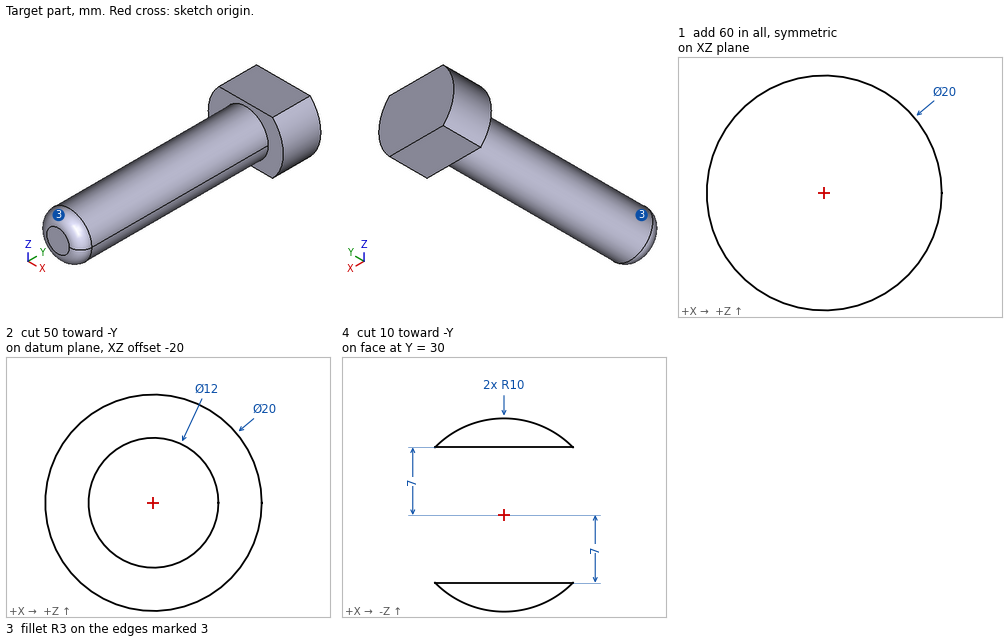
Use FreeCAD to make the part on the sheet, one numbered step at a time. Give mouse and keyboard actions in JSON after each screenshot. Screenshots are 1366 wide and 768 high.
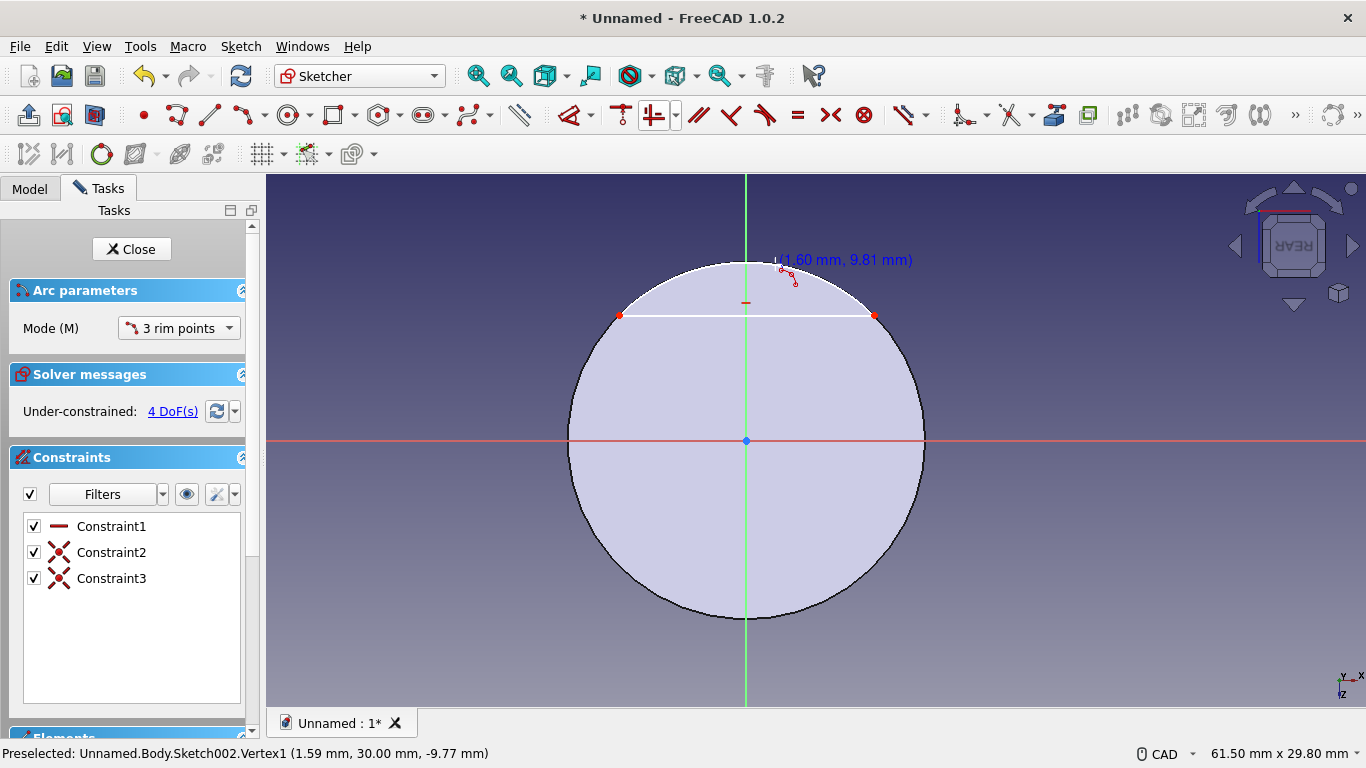
{"action": "left_click", "coordinate": [210, 116]}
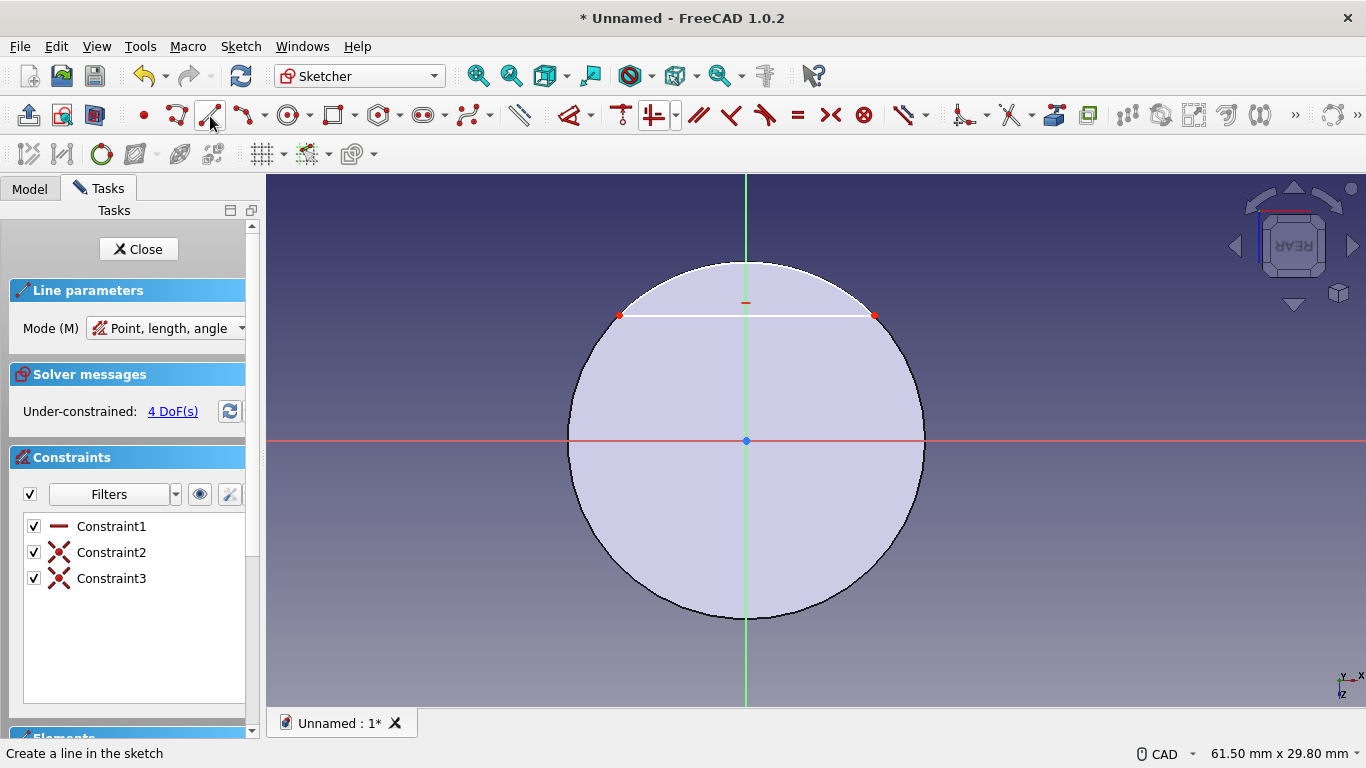
{"action": "left_click", "coordinate": [874, 566]}
{"action": "left_click", "coordinate": [619, 566]}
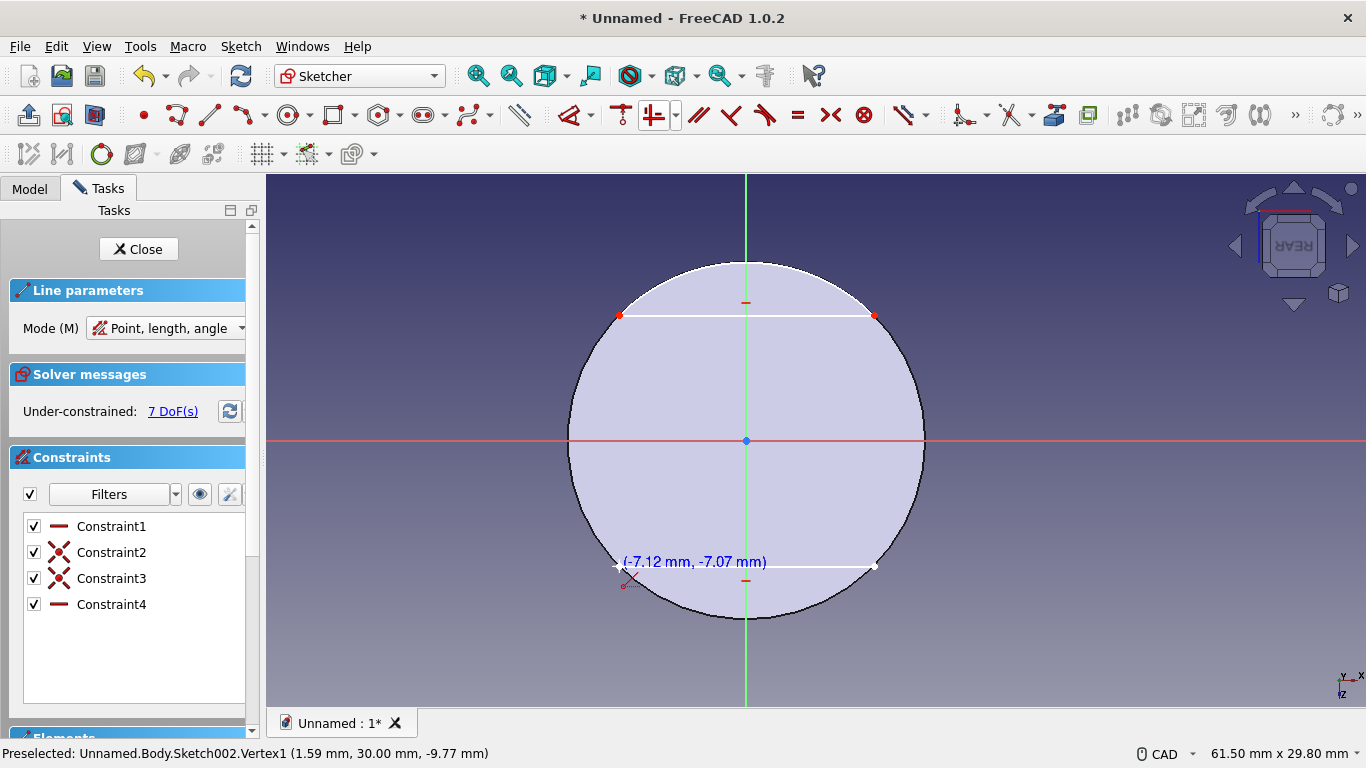
{"action": "key", "text": "g 3 a"}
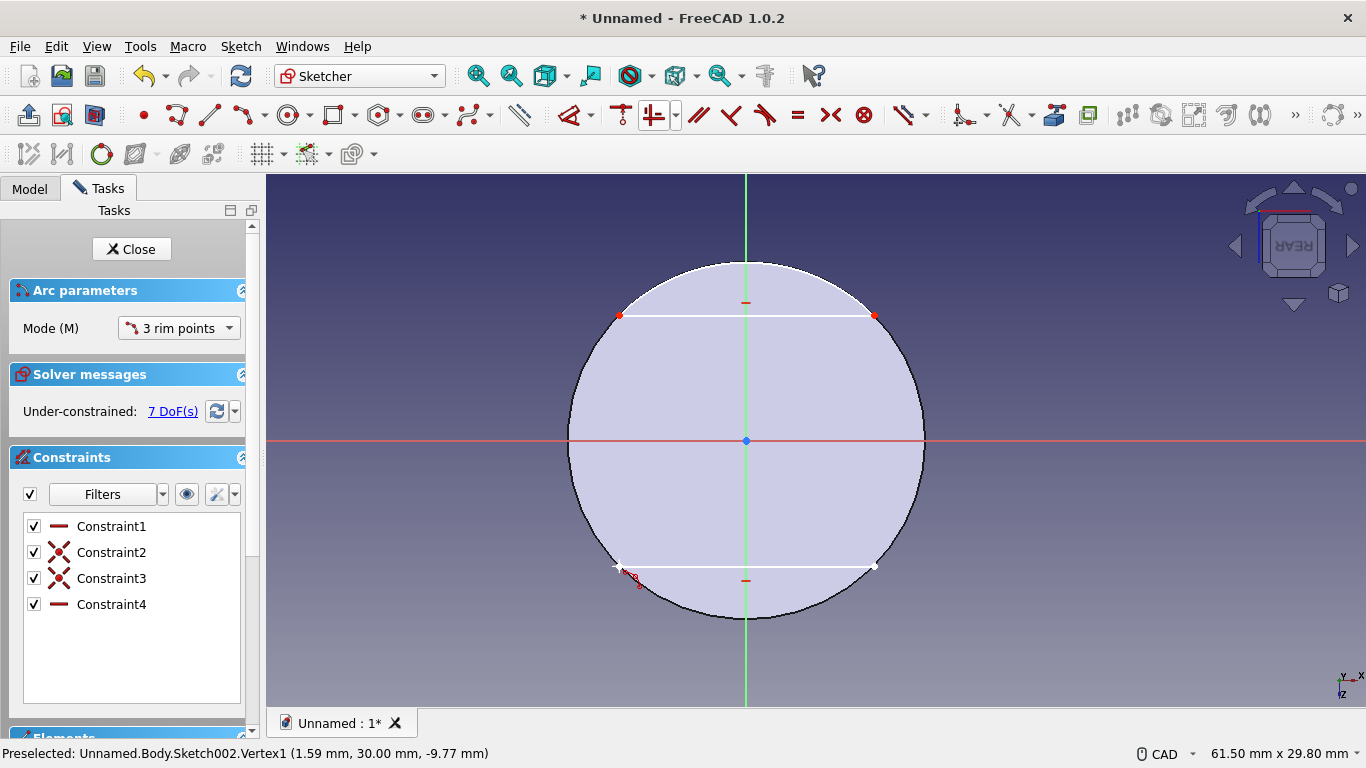
{"action": "left_click", "coordinate": [619, 567]}
{"action": "left_click", "coordinate": [874, 567]}
{"action": "left_click", "coordinate": [718, 617]}
{"action": "key", "text": "Escape"}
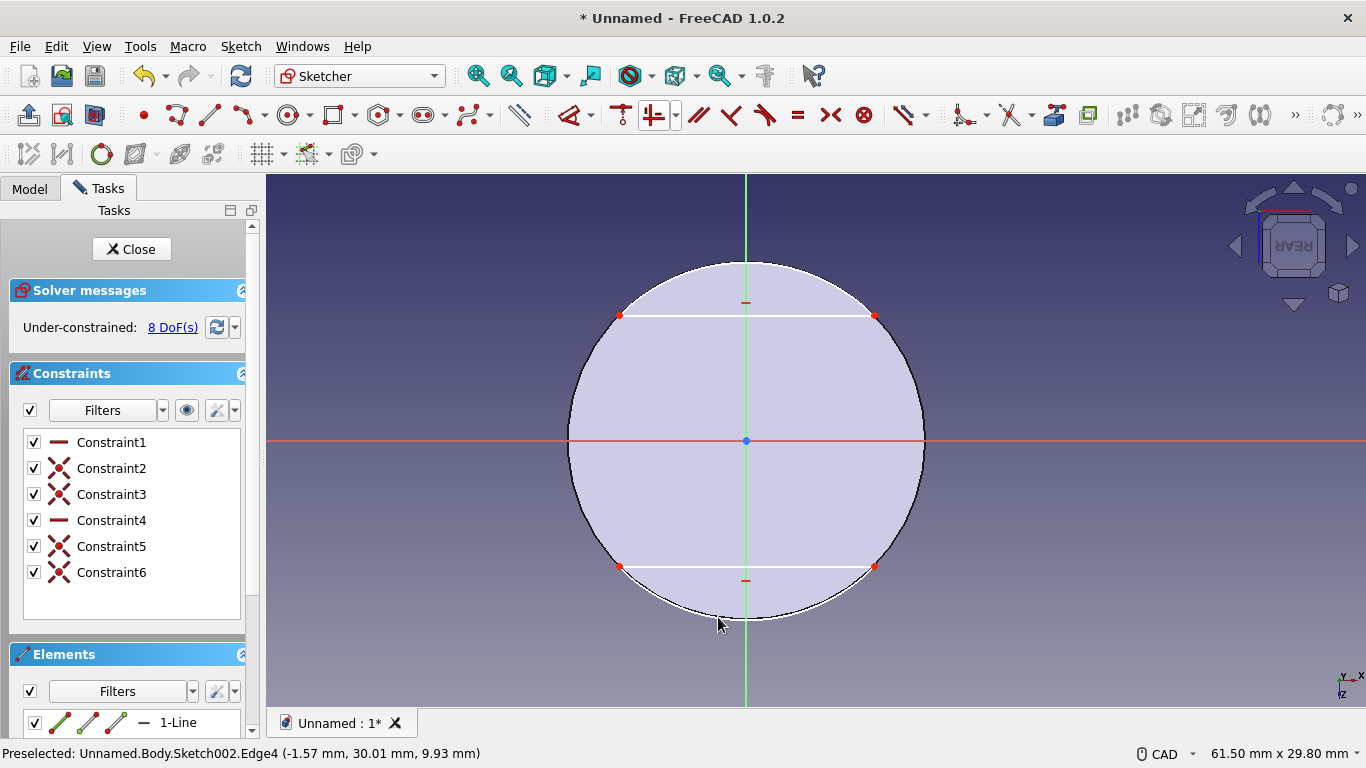
{"action": "left_click", "coordinate": [802, 272]}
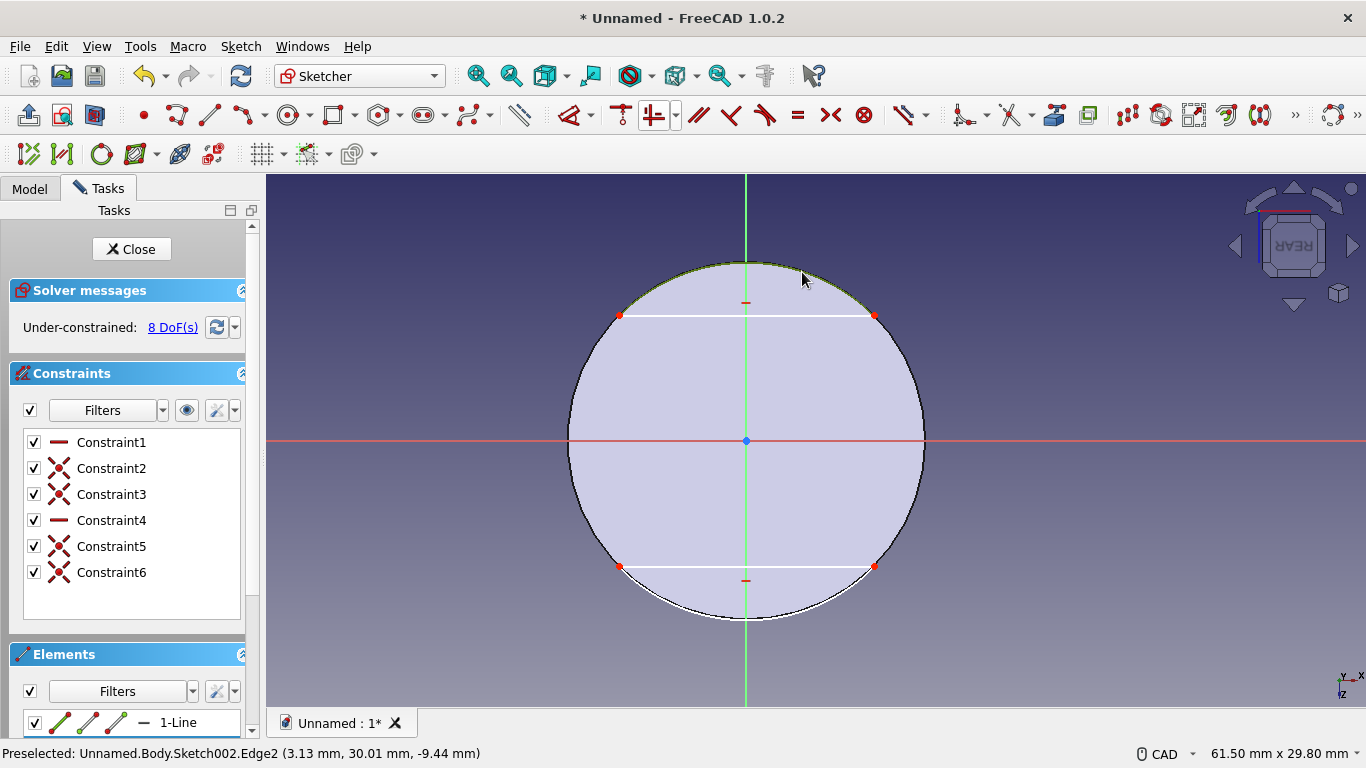
{"action": "left_click", "coordinate": [691, 611]}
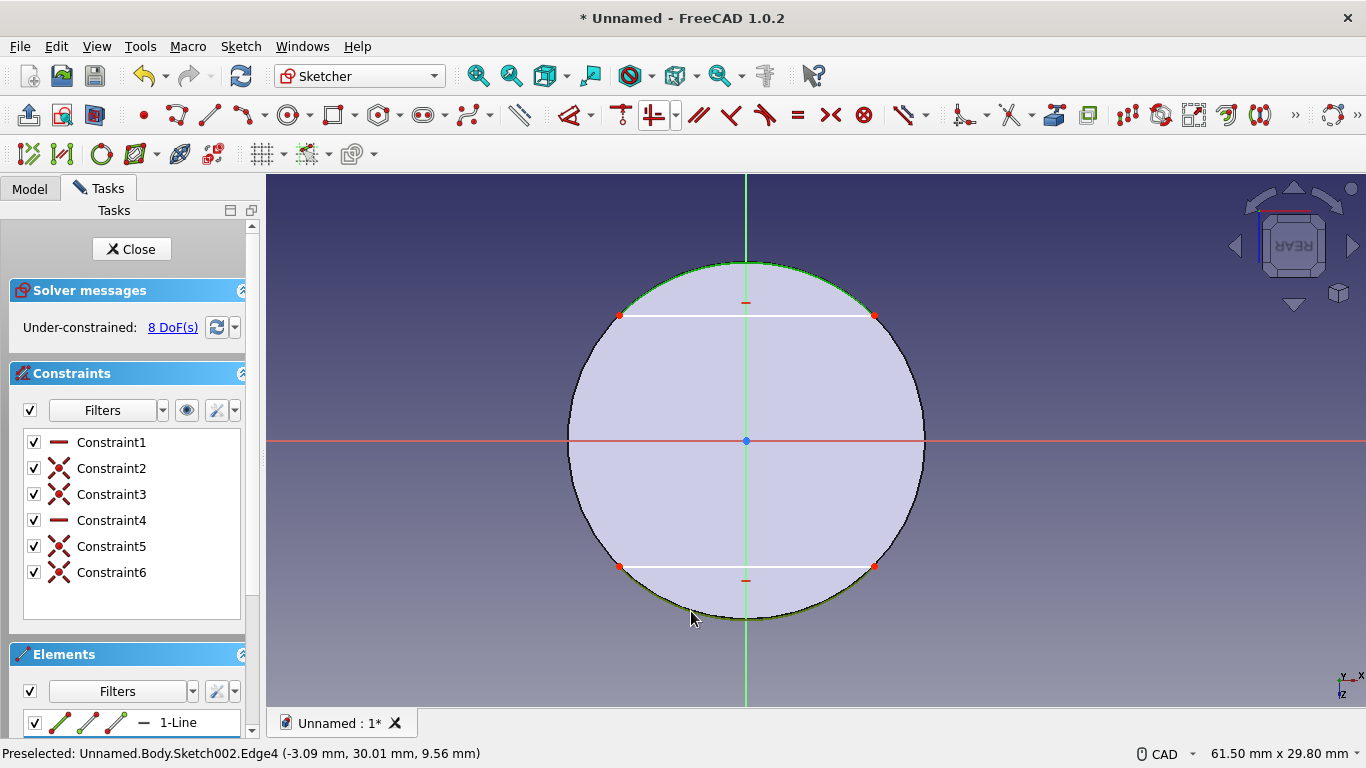
{"action": "key", "text": "c"}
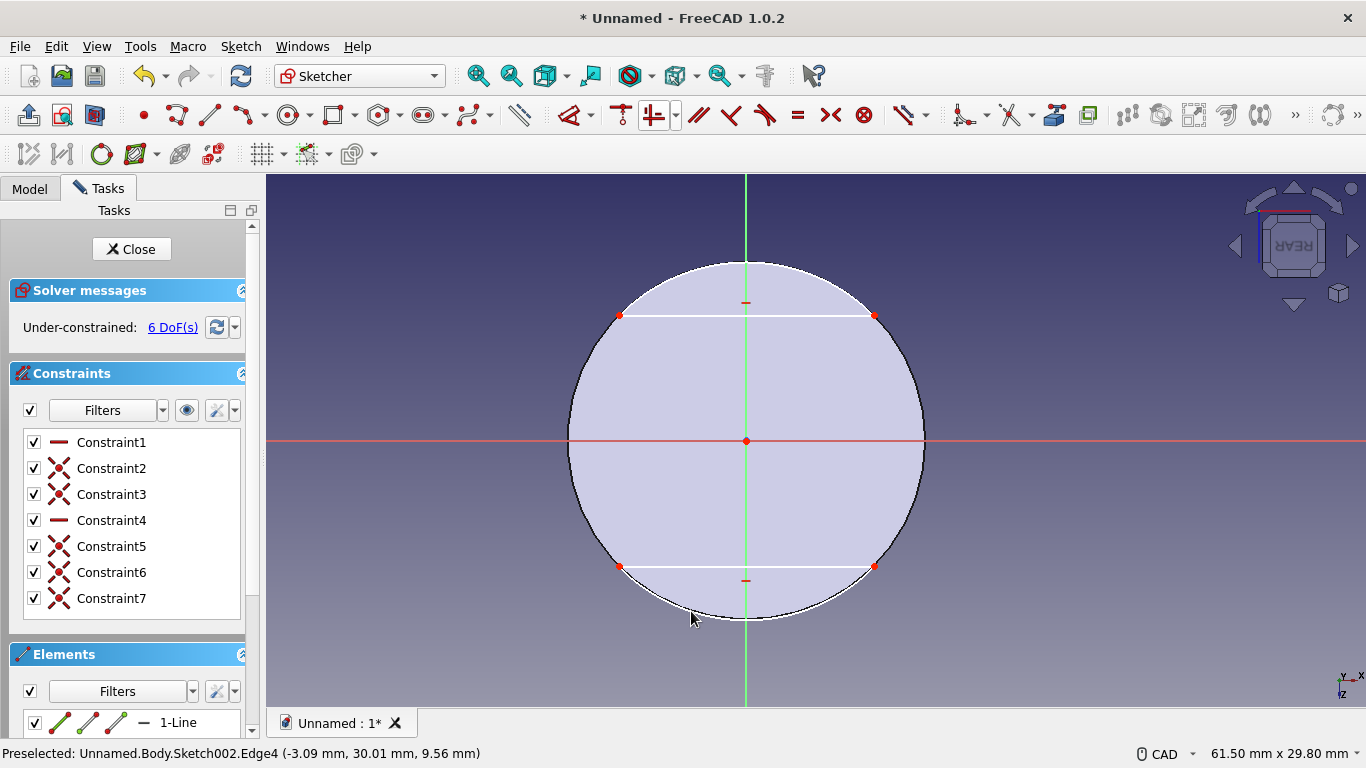
{"action": "left_click_drag", "start_coordinate": [736, 430], "coordinate": [757, 451]}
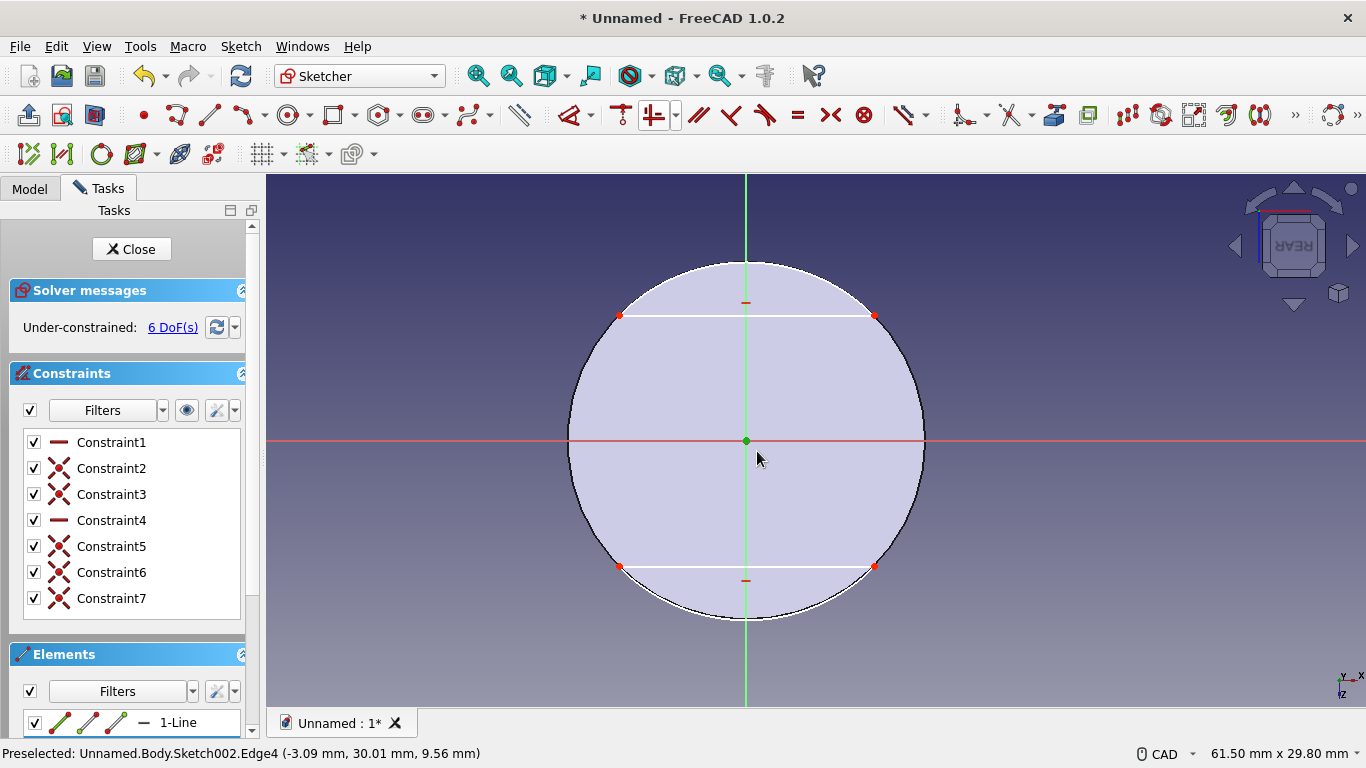
{"action": "left_click", "coordinate": [621, 116]}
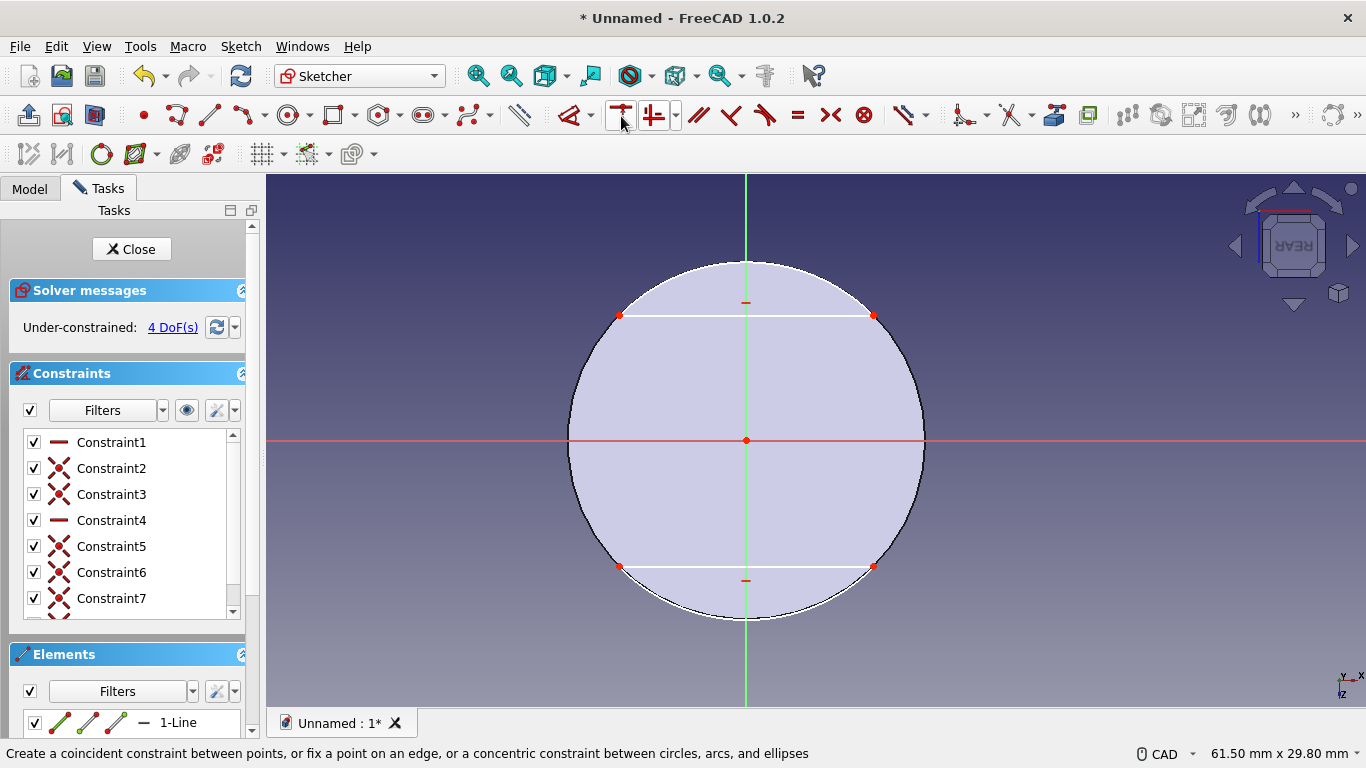
{"action": "left_click", "coordinate": [802, 271]}